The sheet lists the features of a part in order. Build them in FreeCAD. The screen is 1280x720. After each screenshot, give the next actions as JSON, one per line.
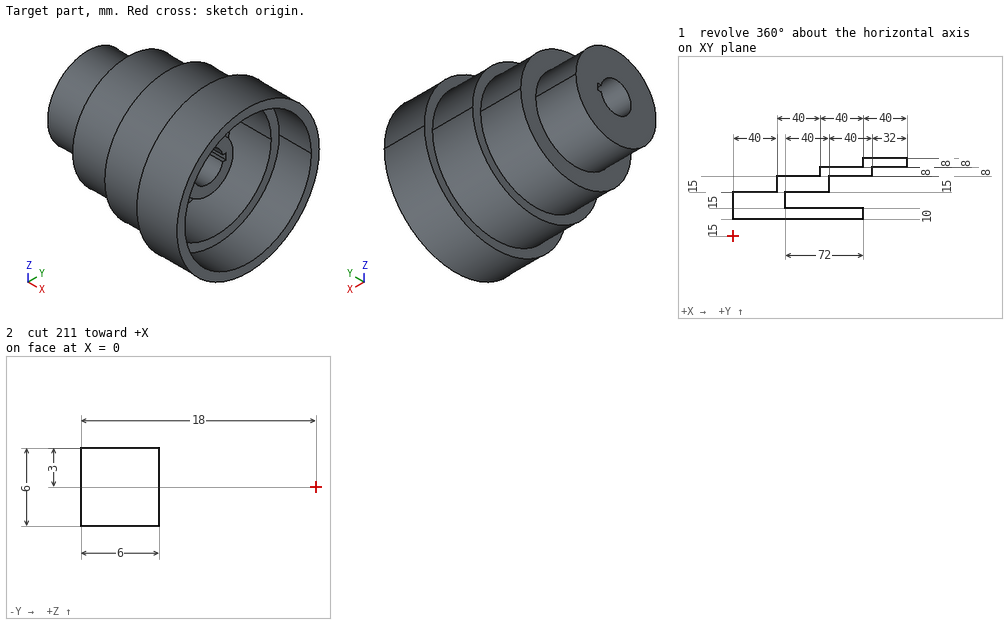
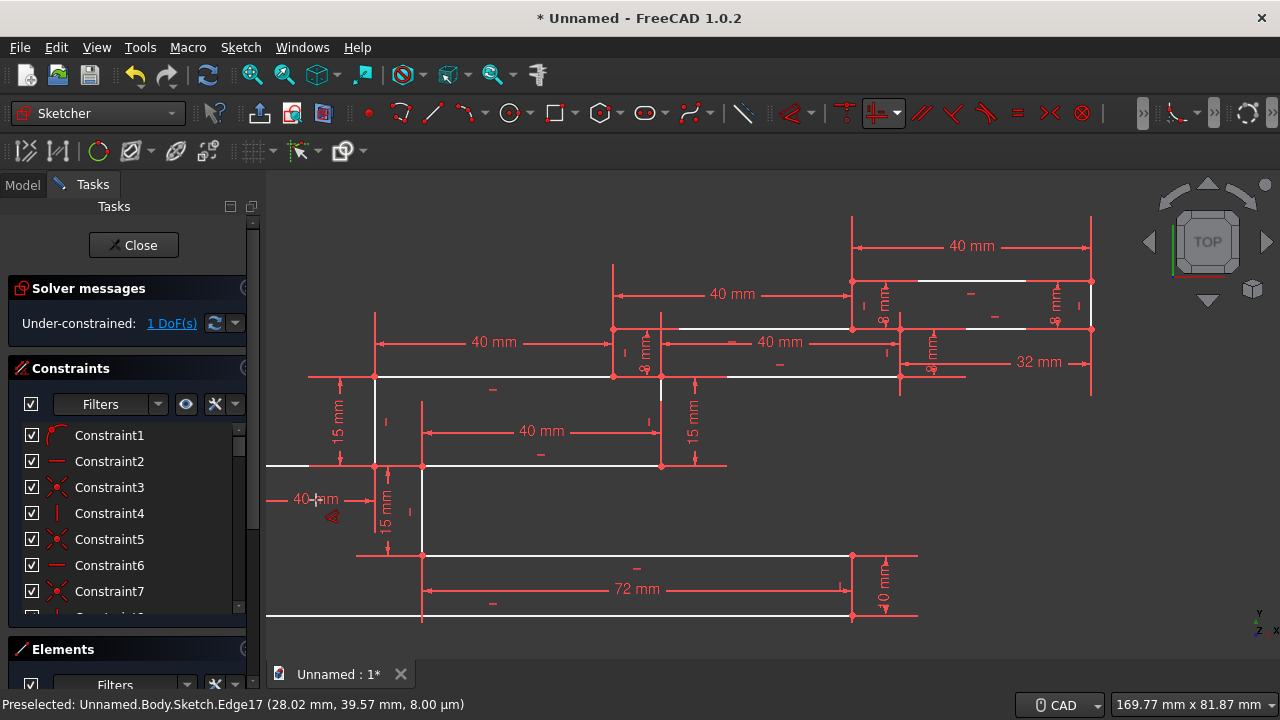
{"action": "scroll", "coordinate": [815, 322], "scroll_direction": "down", "scroll_amount": 3}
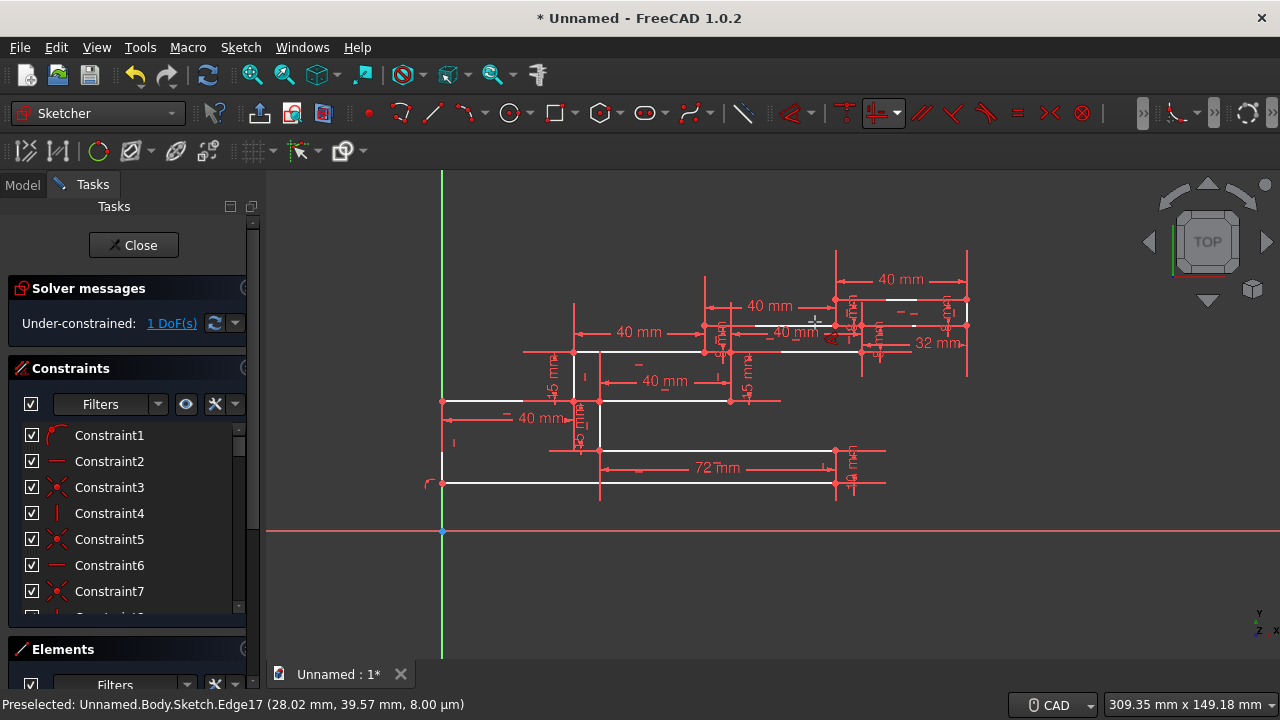
{"action": "left_click", "coordinate": [442, 483]}
{"action": "left_click", "coordinate": [408, 507]}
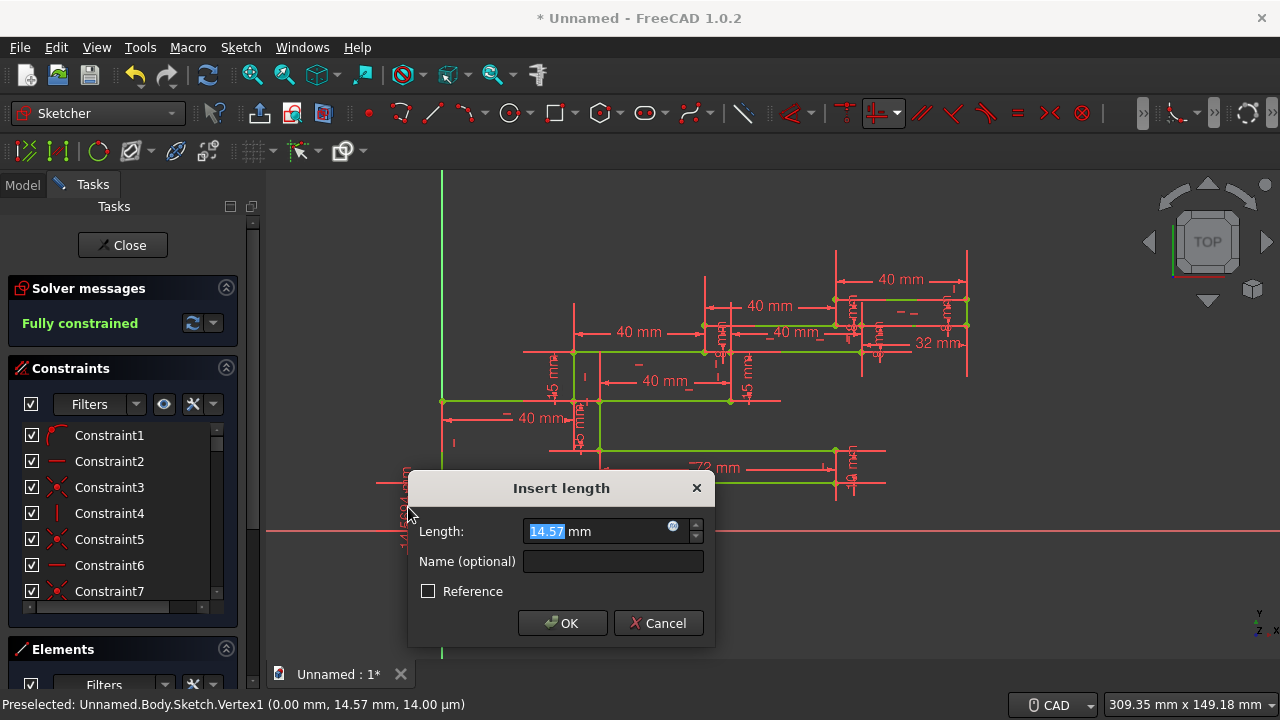
{"action": "type", "text": "15"}
{"action": "key", "text": "Return"}
{"action": "key", "text": "Escape"}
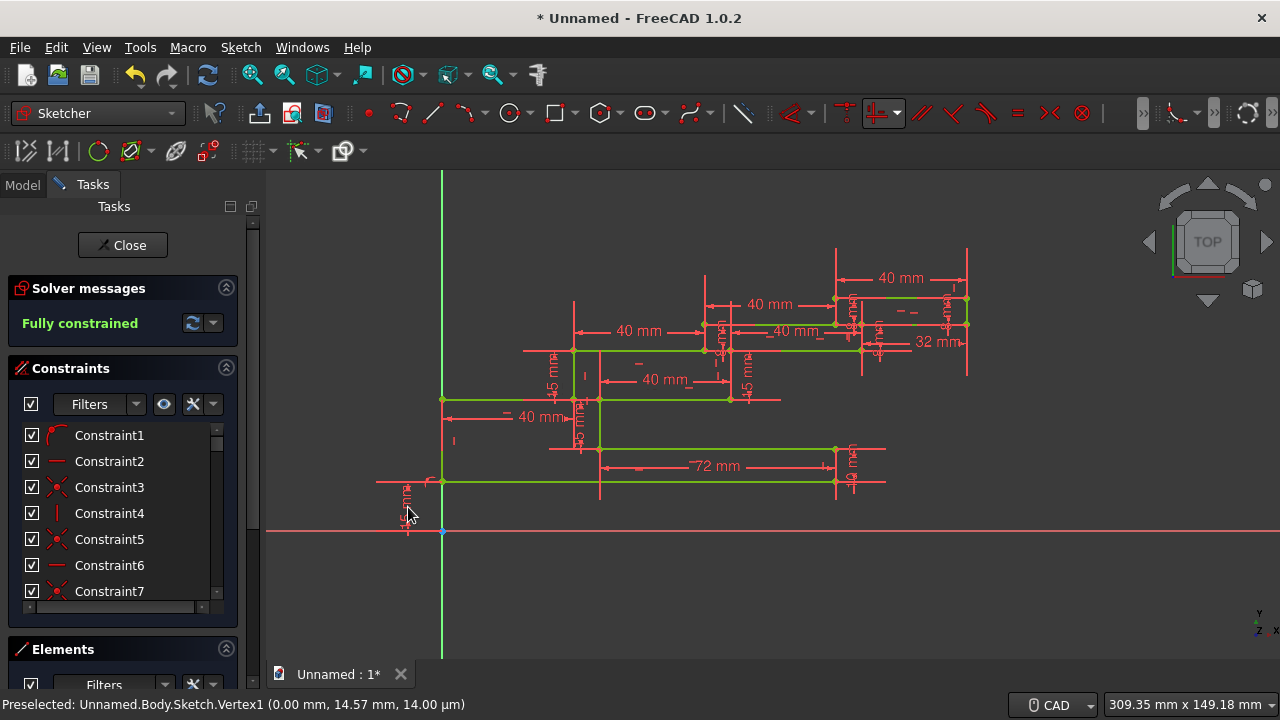
{"action": "left_click", "coordinate": [123, 245]}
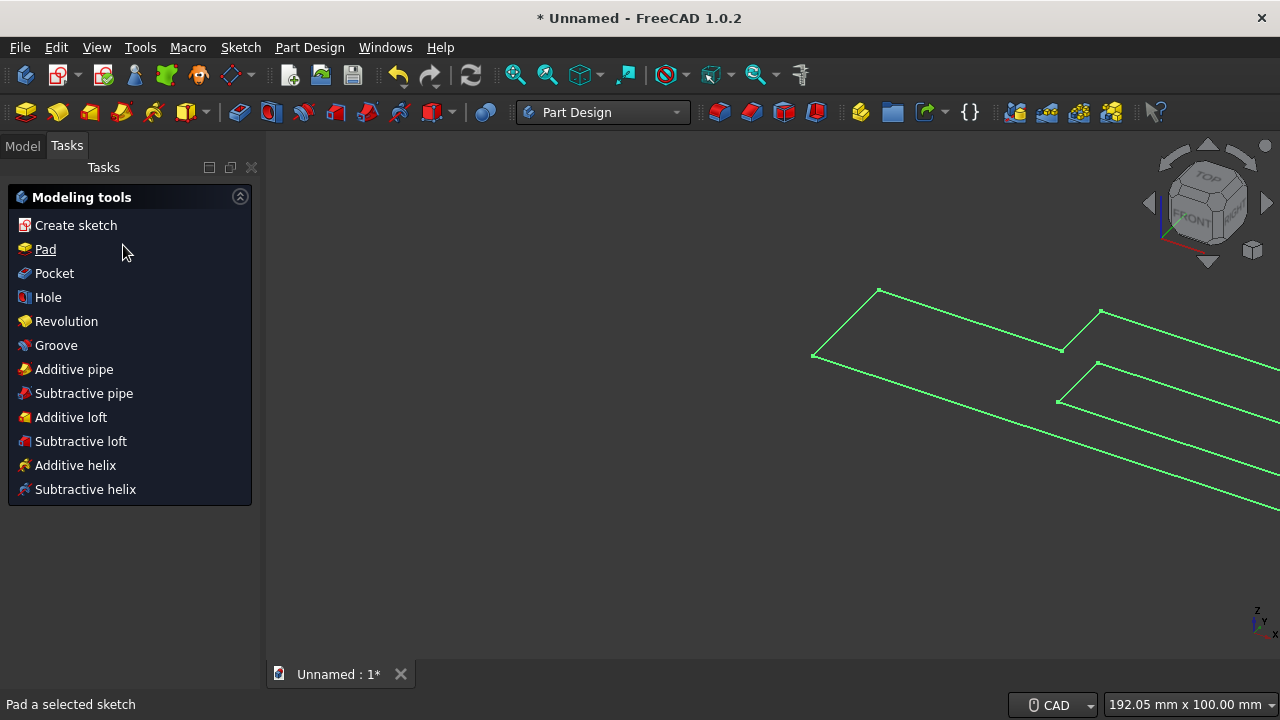
{"action": "left_click", "coordinate": [58, 112]}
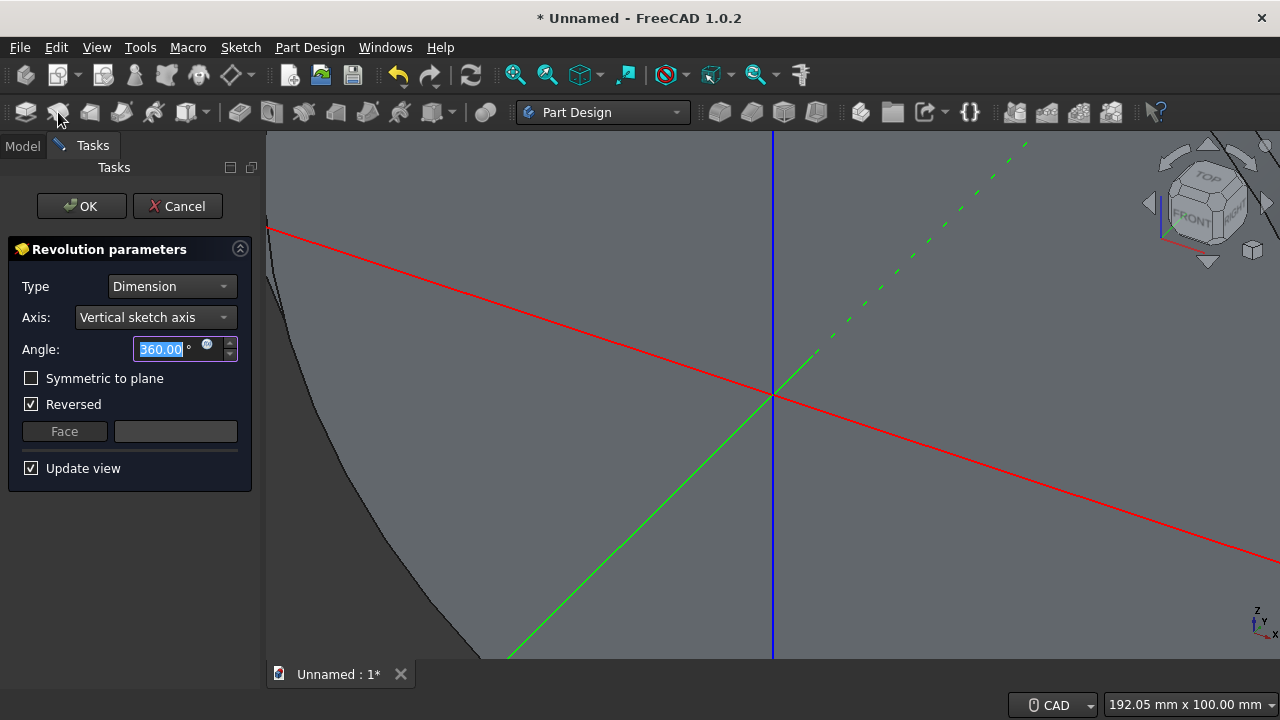
{"action": "left_click", "coordinate": [156, 318]}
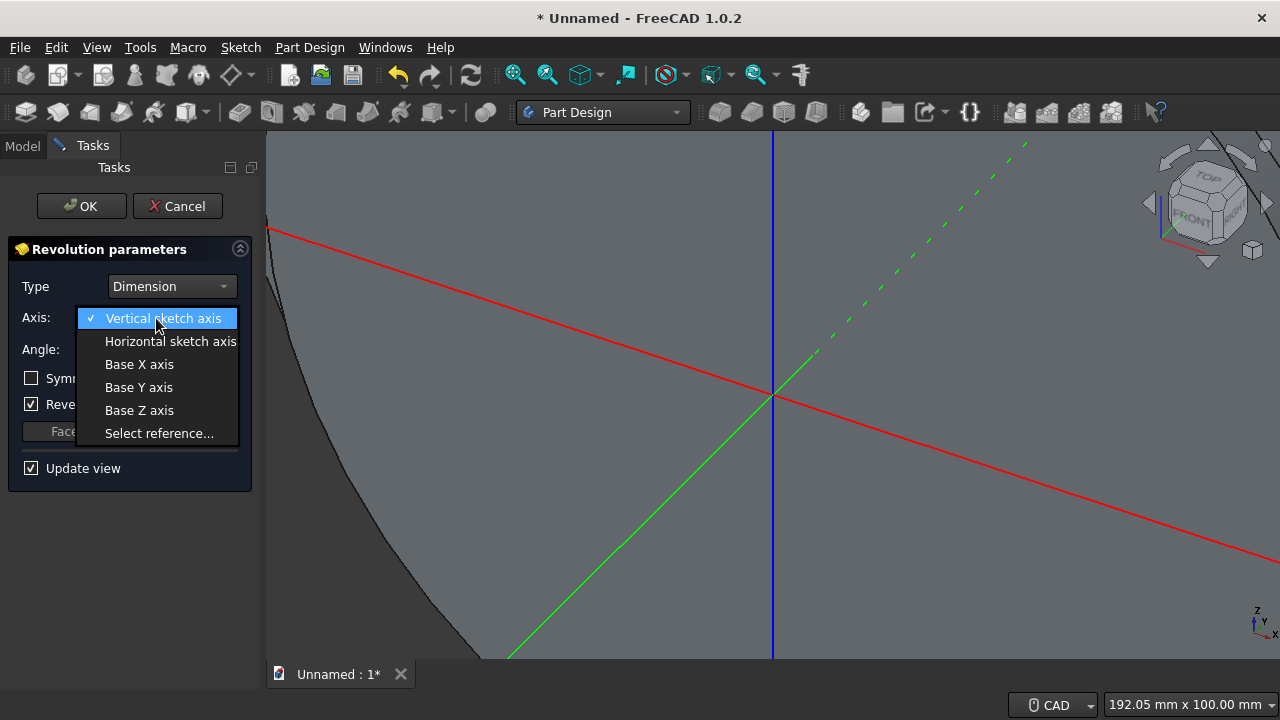
{"action": "left_click", "coordinate": [156, 342]}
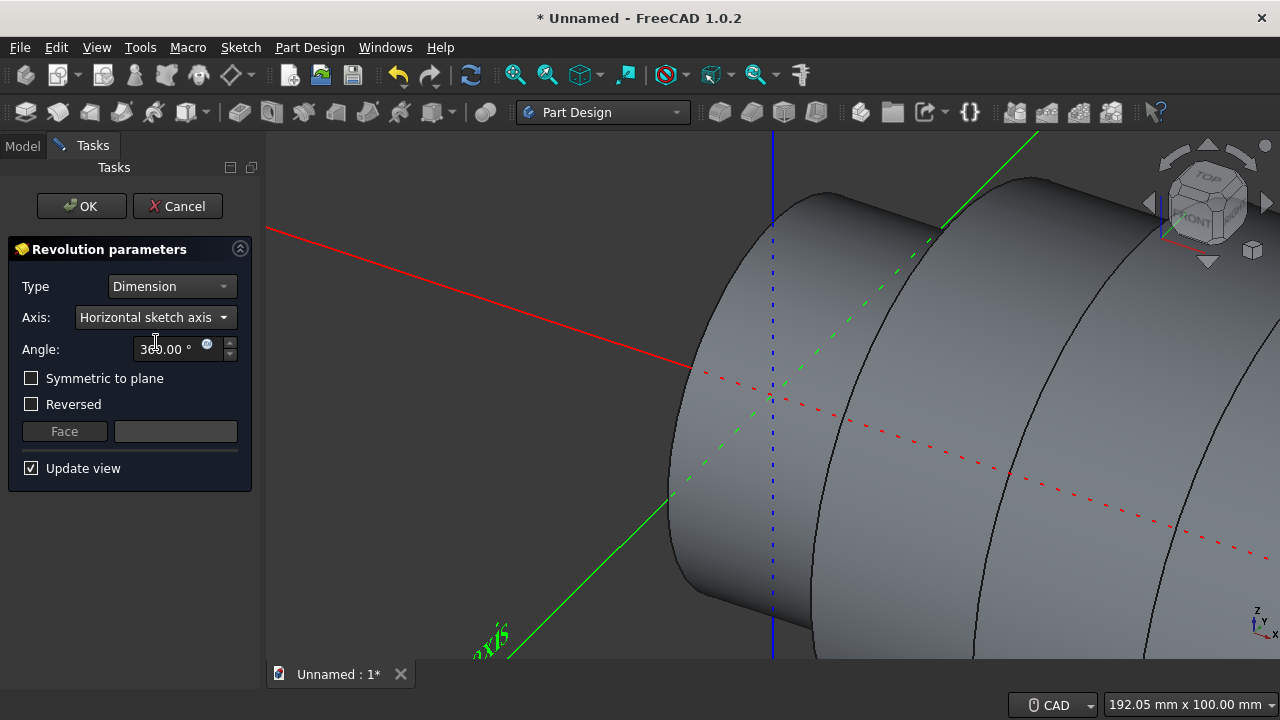
{"action": "left_click", "coordinate": [82, 206]}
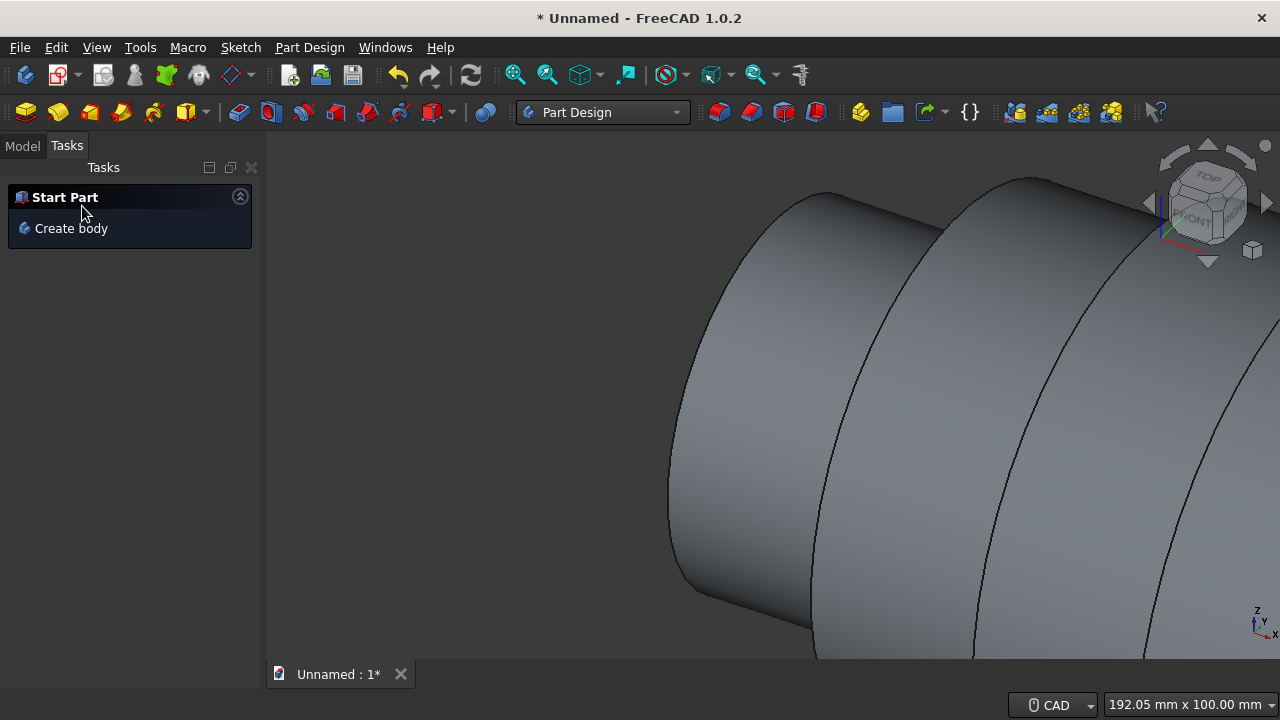
{"action": "key", "text": "v f"}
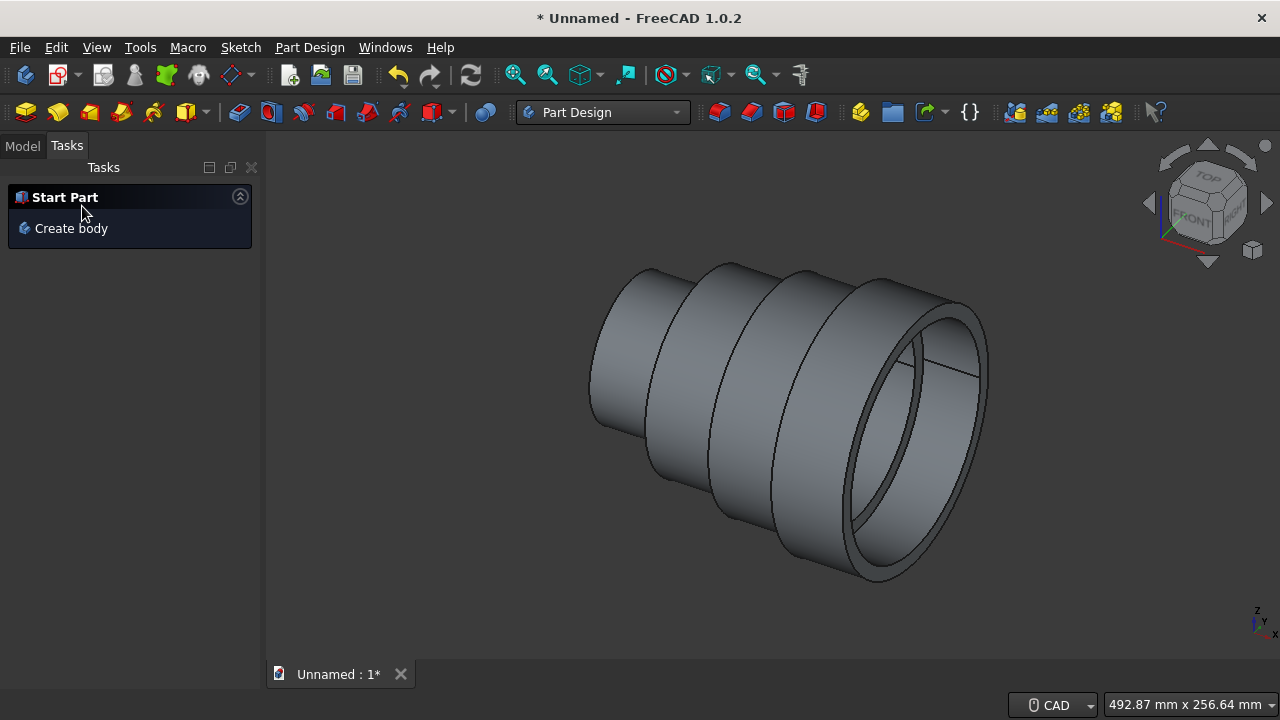
{"action": "key", "text": "6"}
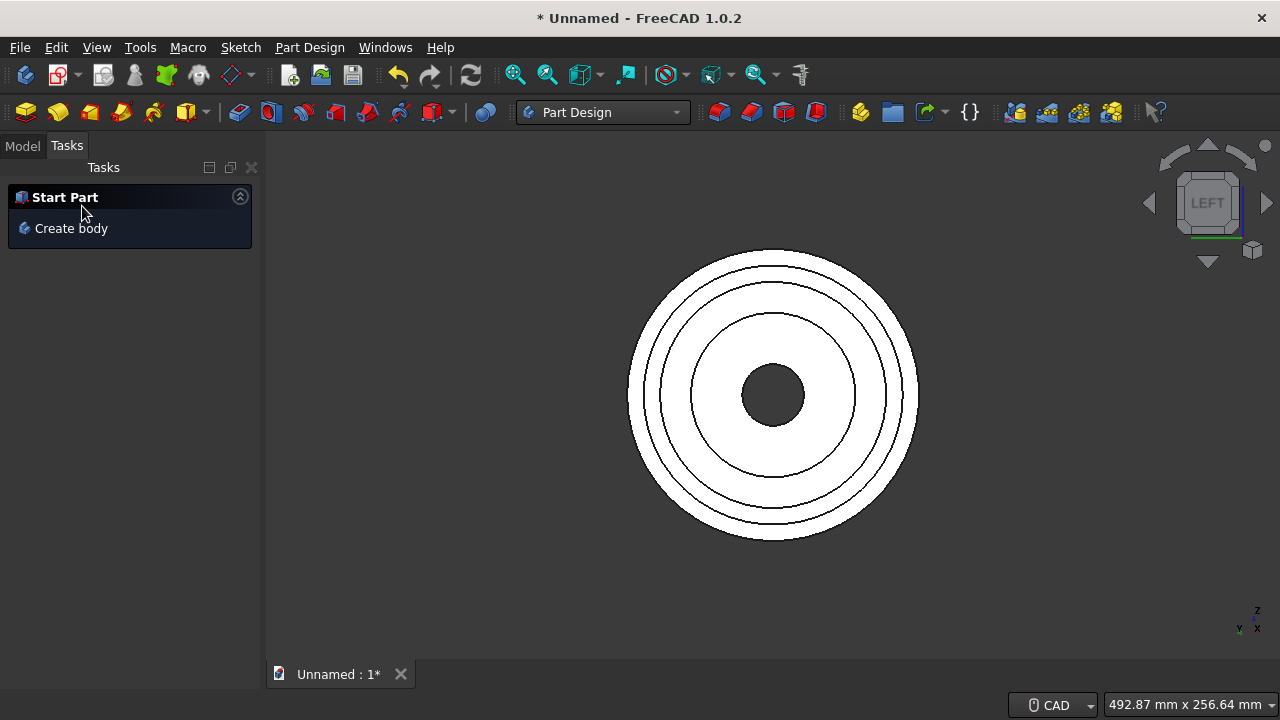
{"action": "left_click", "coordinate": [750, 441]}